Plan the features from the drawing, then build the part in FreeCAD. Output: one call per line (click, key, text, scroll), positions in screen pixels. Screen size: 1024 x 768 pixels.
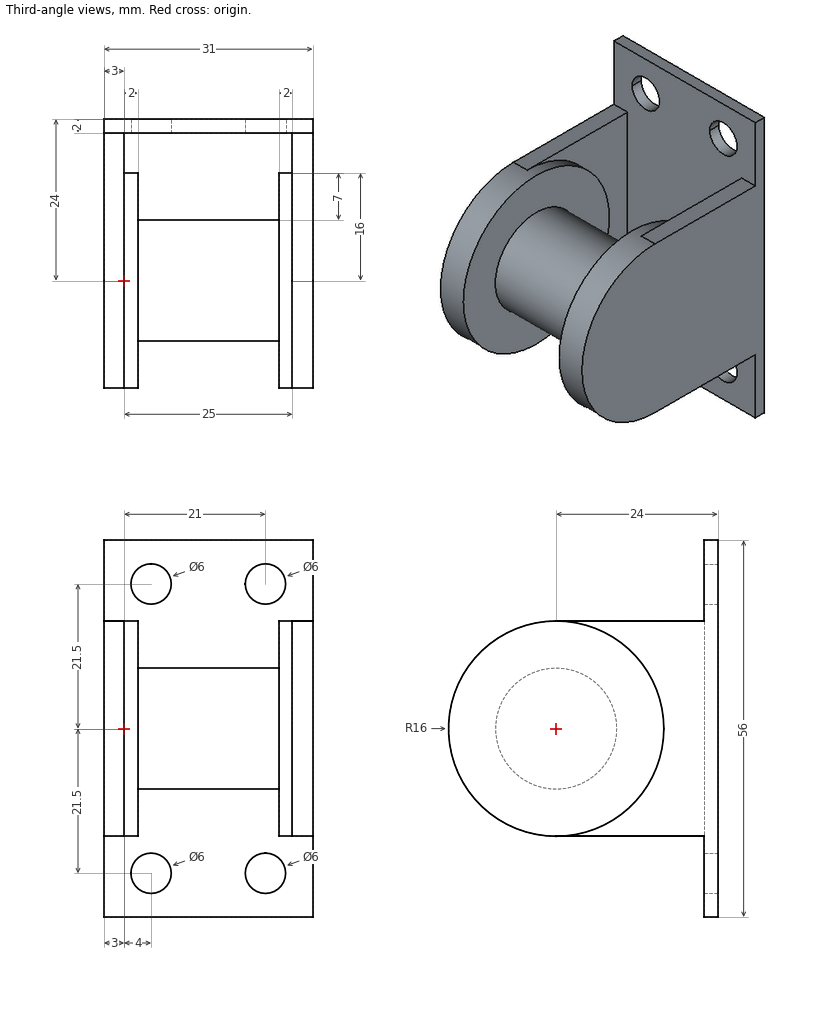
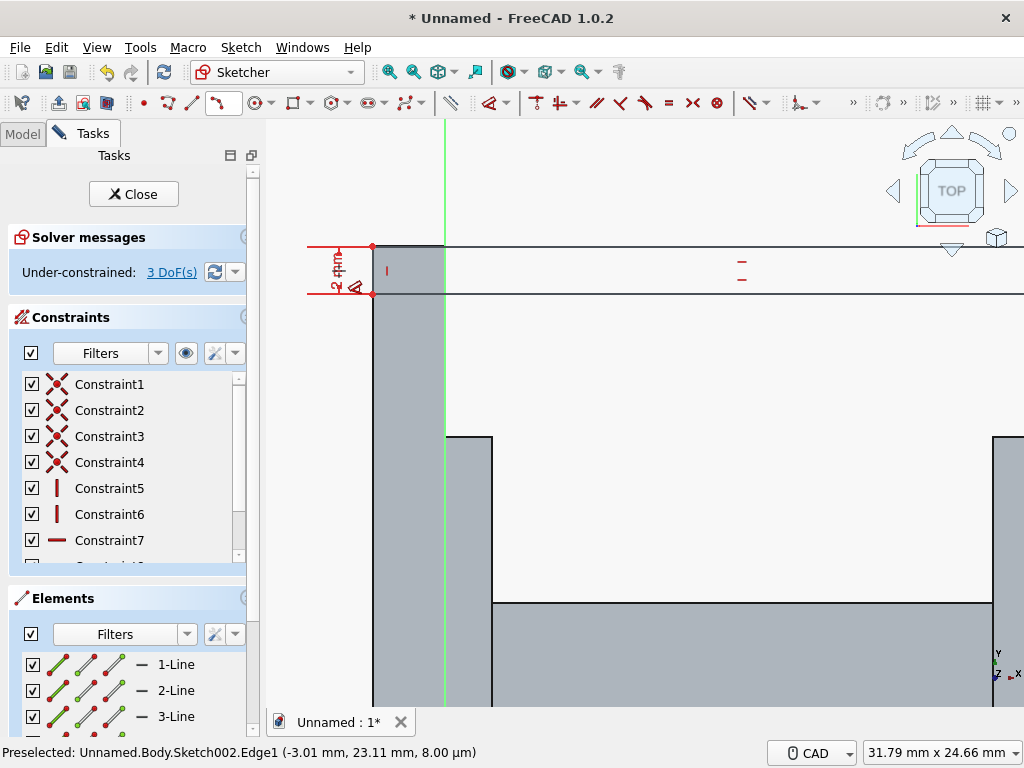
click(595, 294)
click(616, 260)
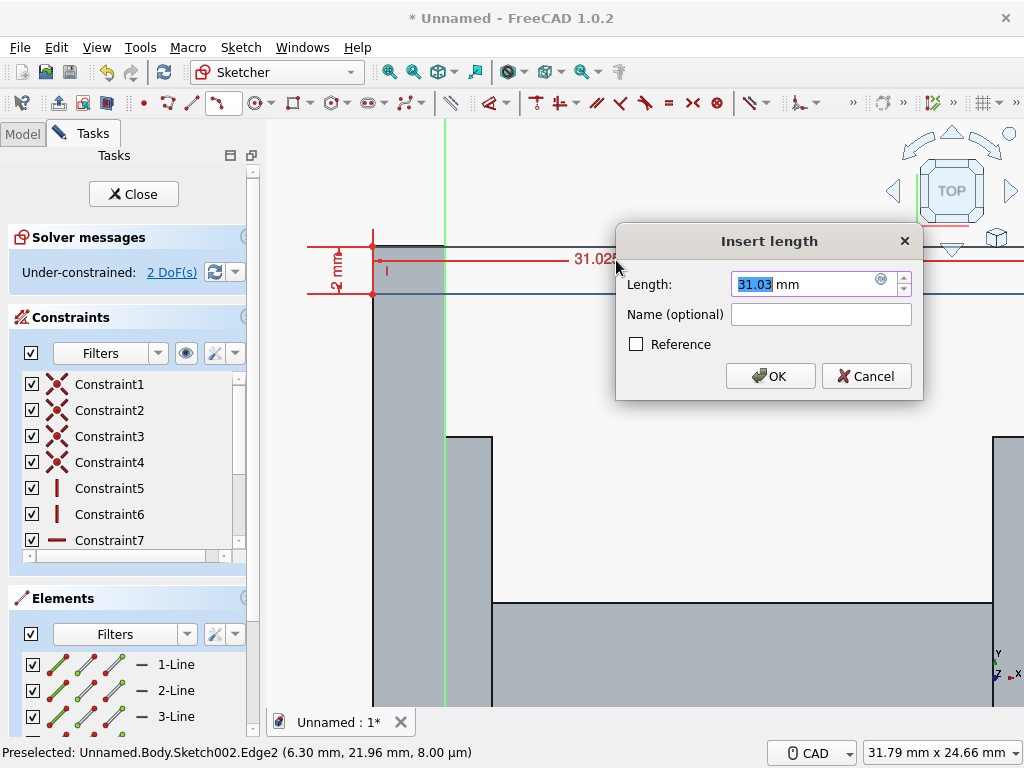
text(31)
key(Return)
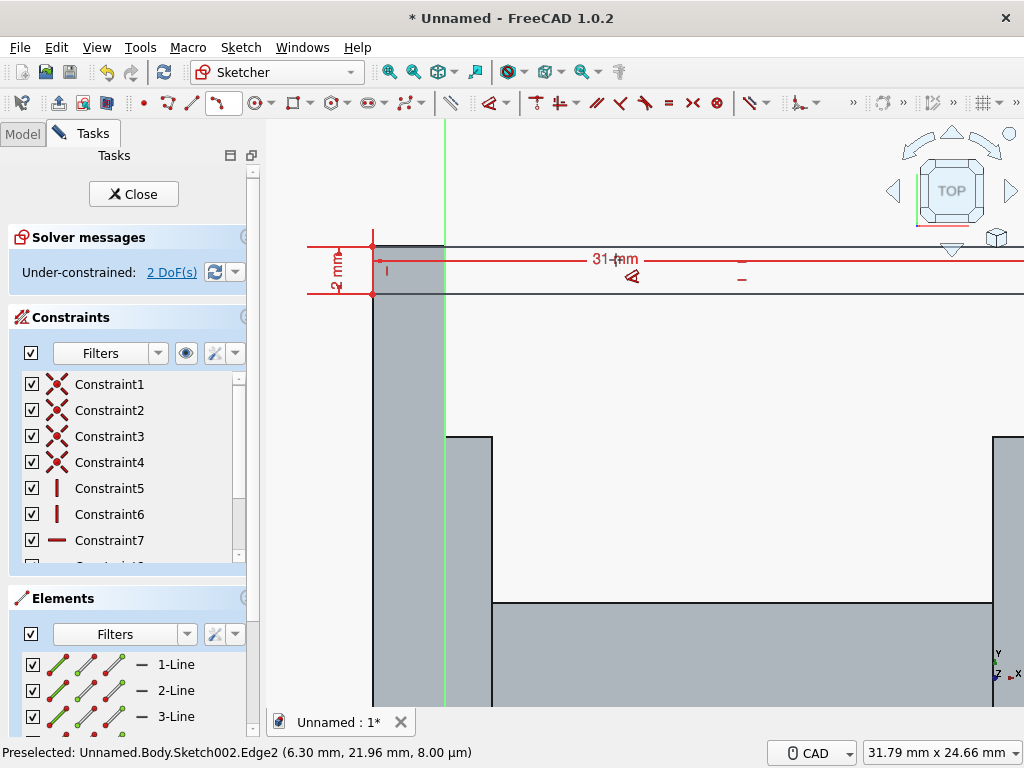
click(373, 247)
click(409, 213)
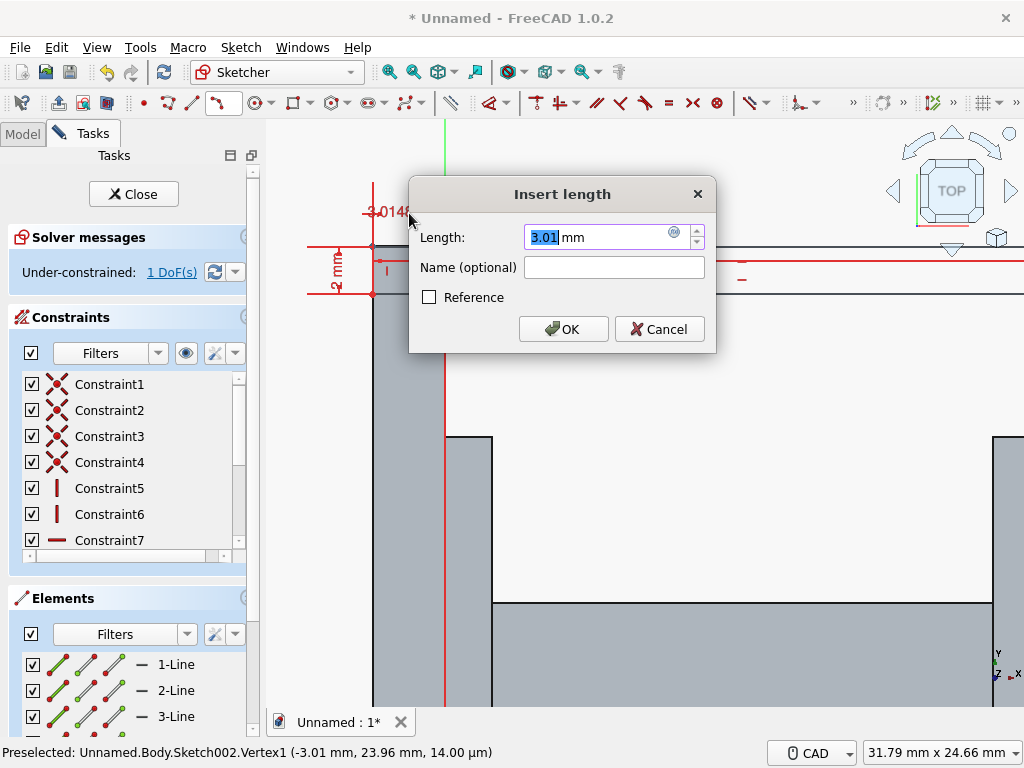
text(3)
key(Return)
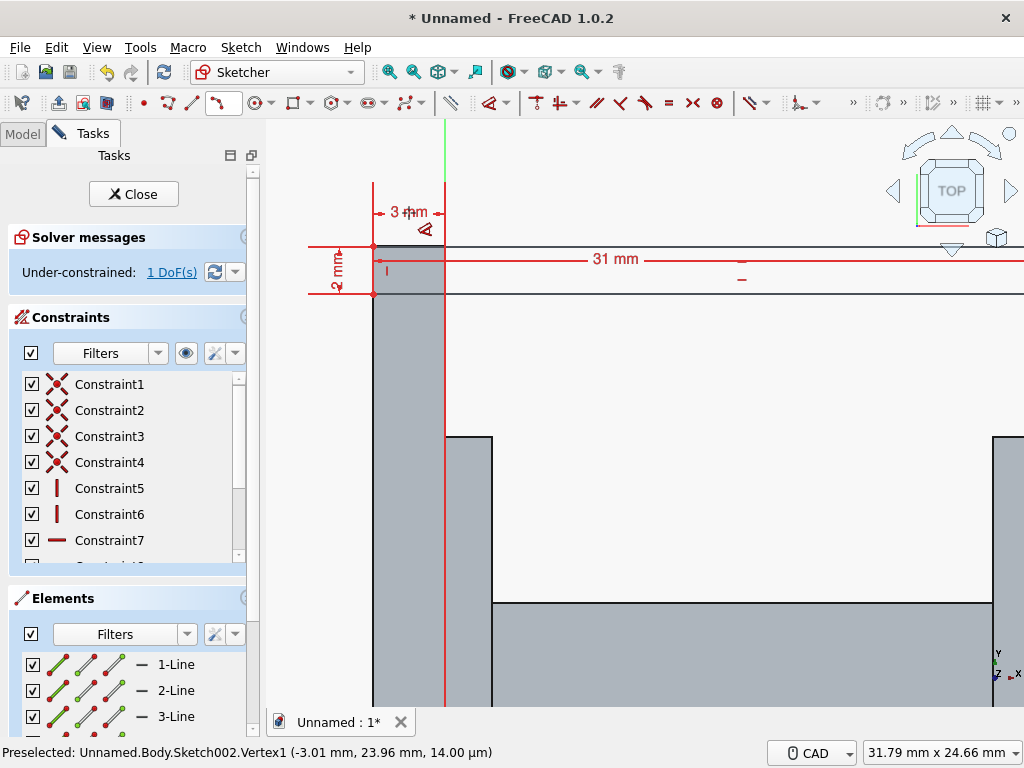
click(373, 247)
click(339, 463)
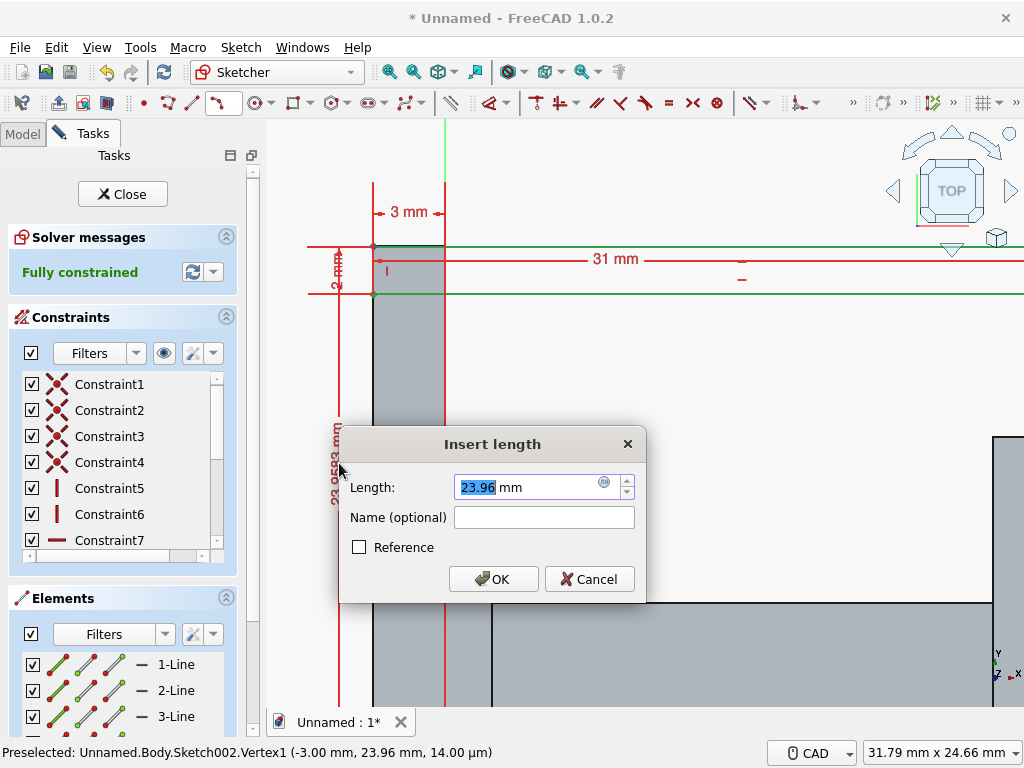
text(24)
key(Return)
key(Escape)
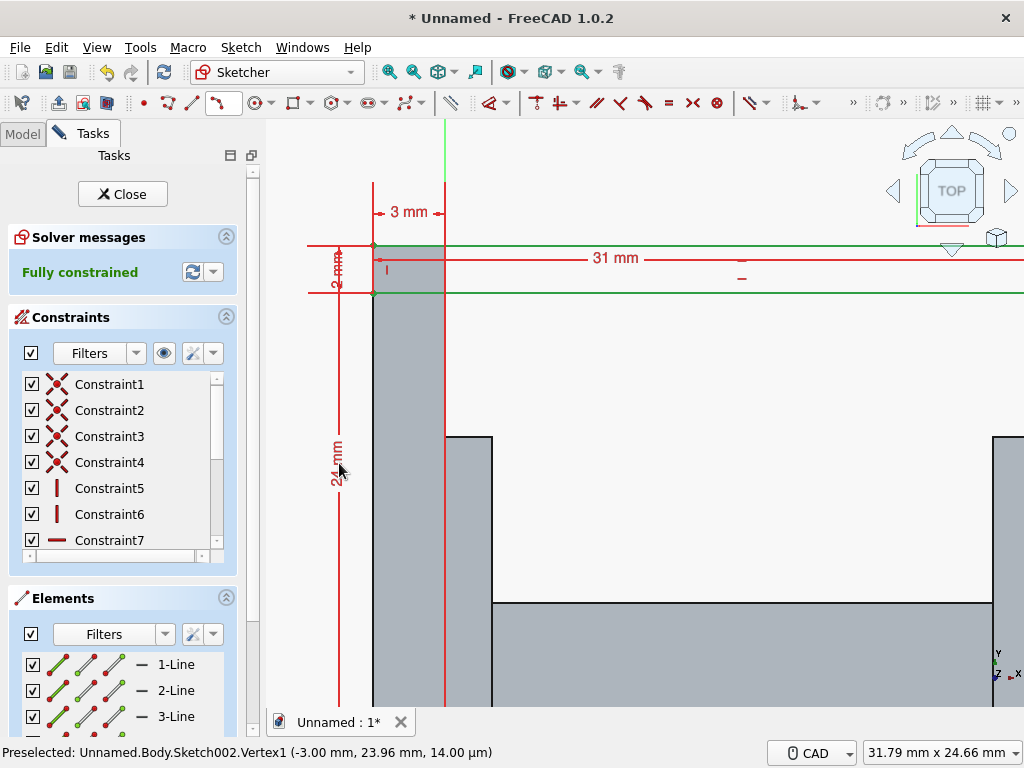
click(123, 194)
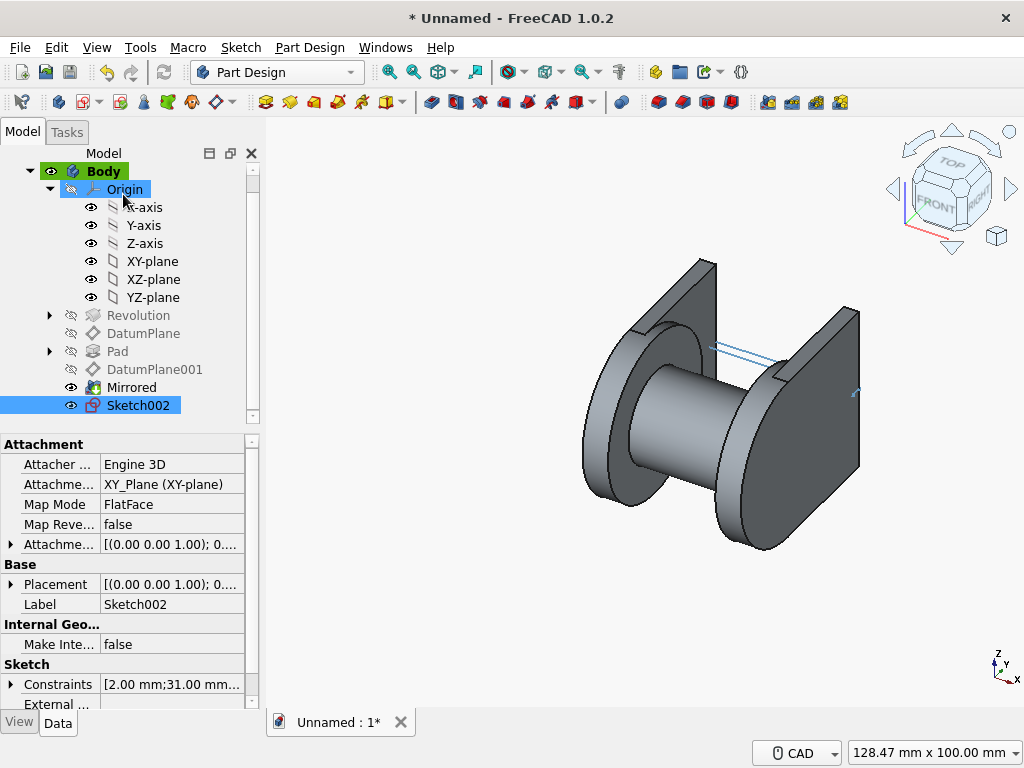
click(266, 102)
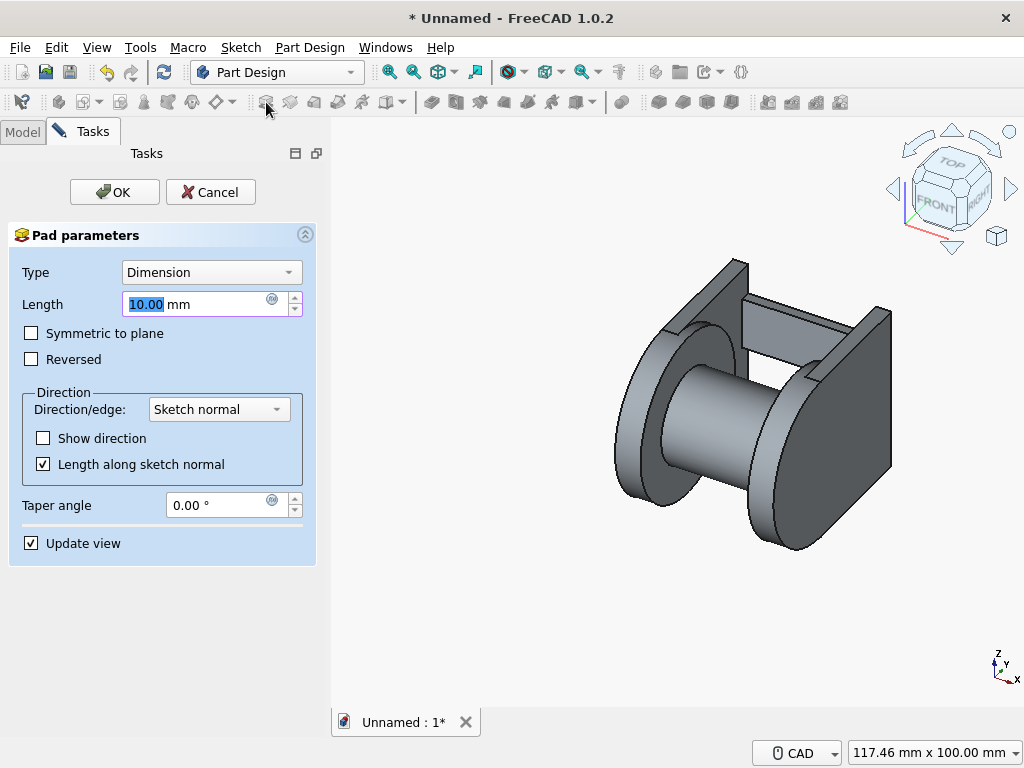
text(56)
key(Tab)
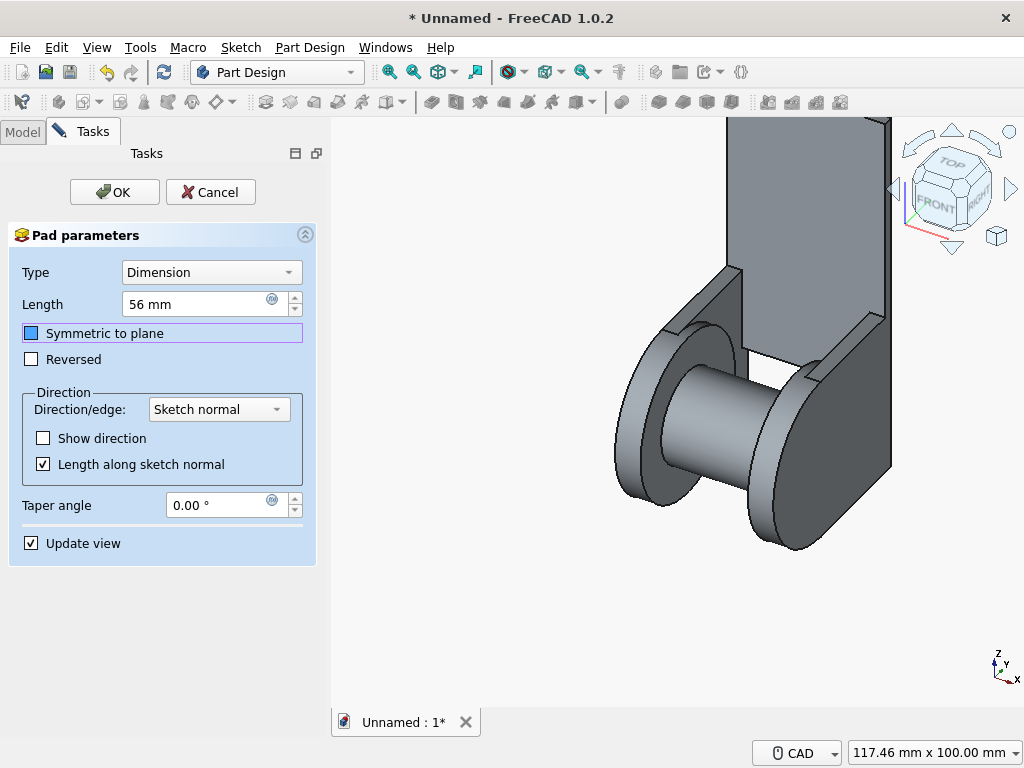
click(30, 333)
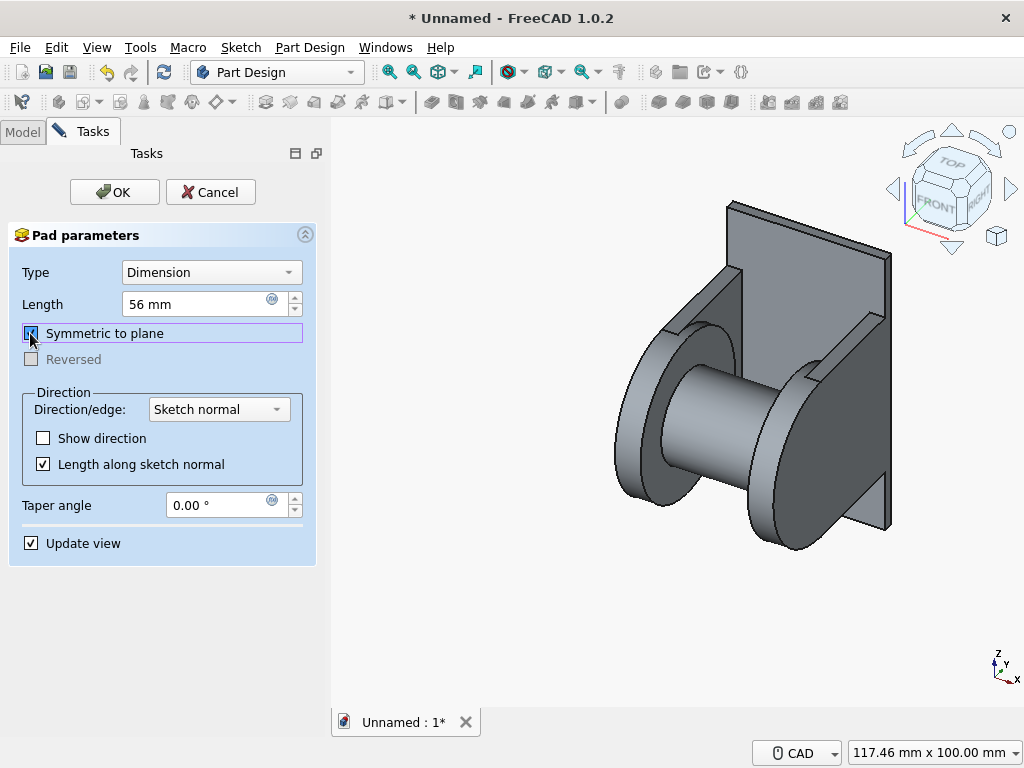
click(115, 192)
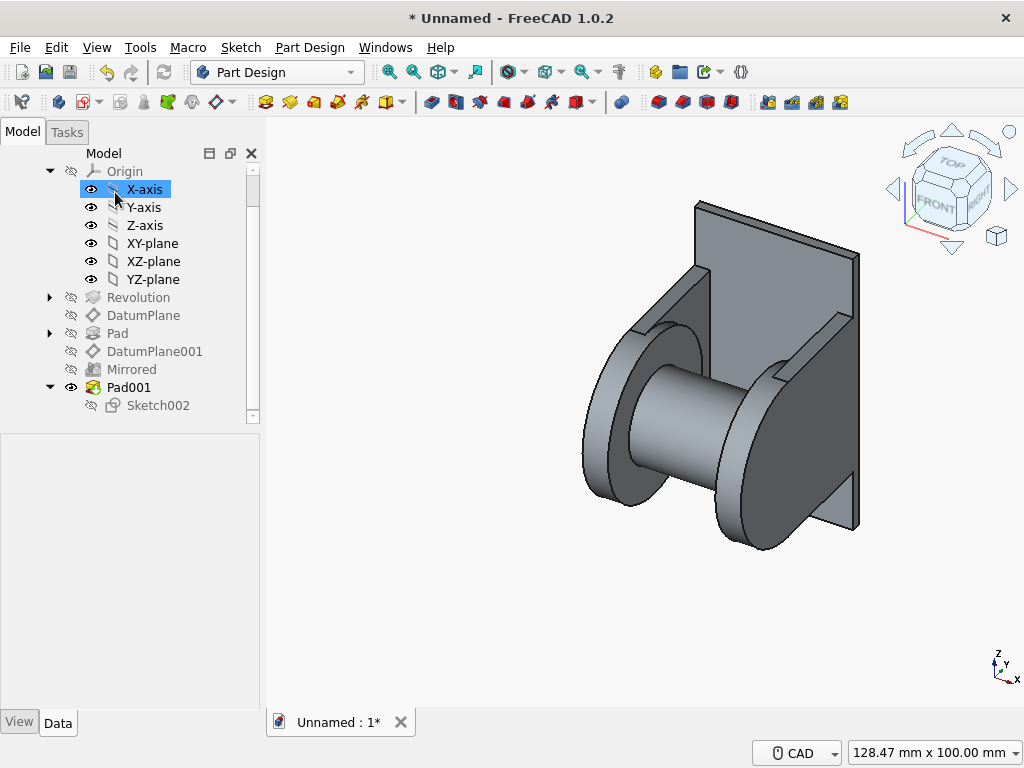
key(4)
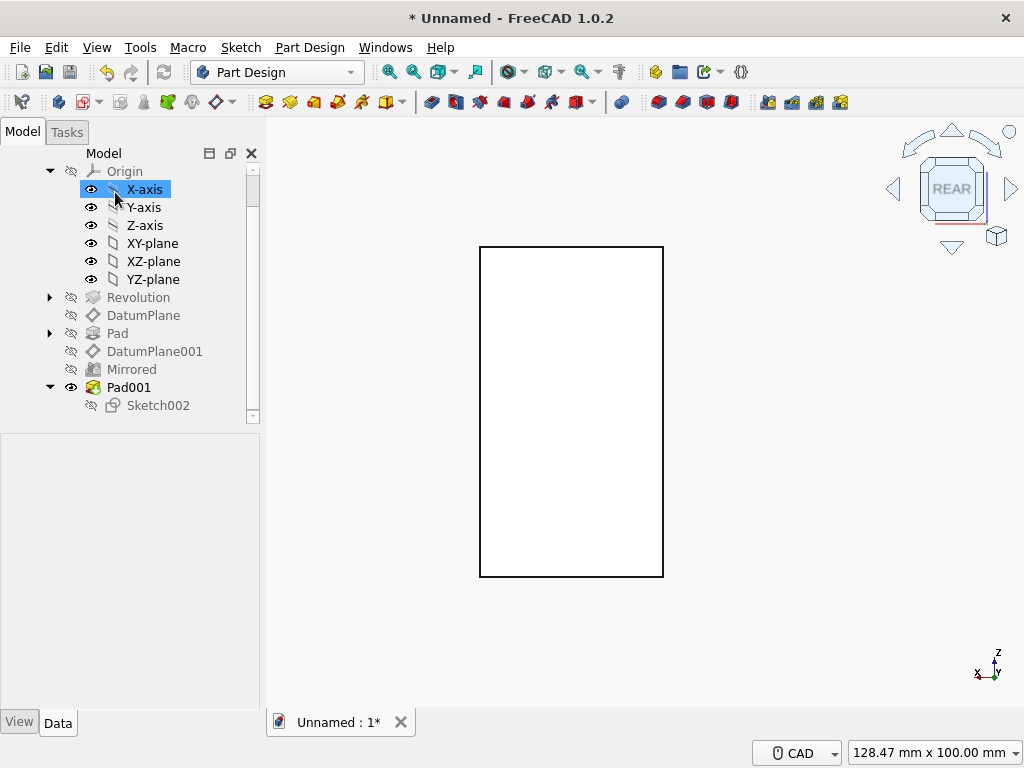
click(571, 364)